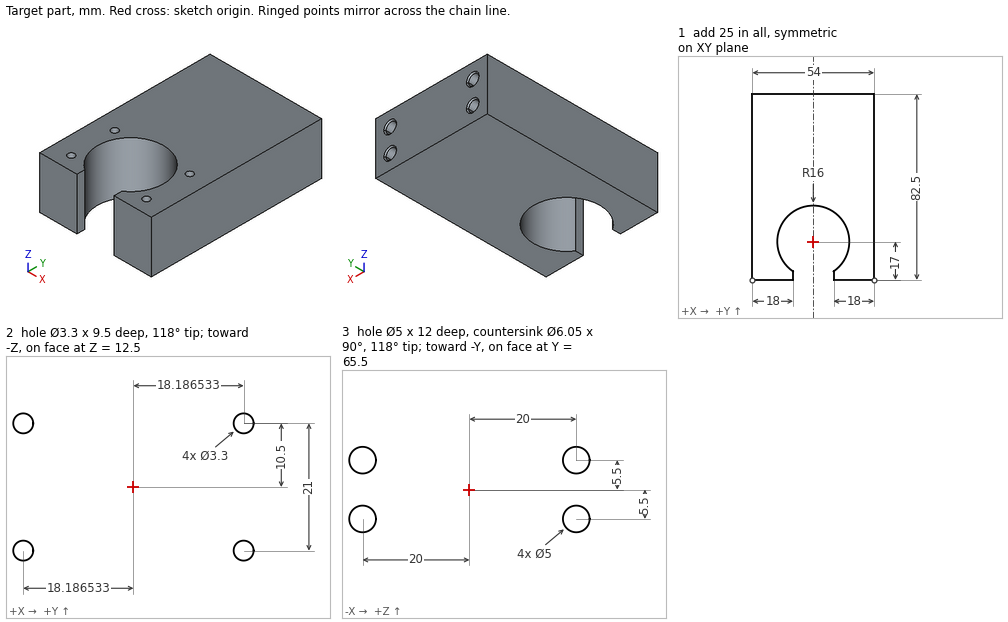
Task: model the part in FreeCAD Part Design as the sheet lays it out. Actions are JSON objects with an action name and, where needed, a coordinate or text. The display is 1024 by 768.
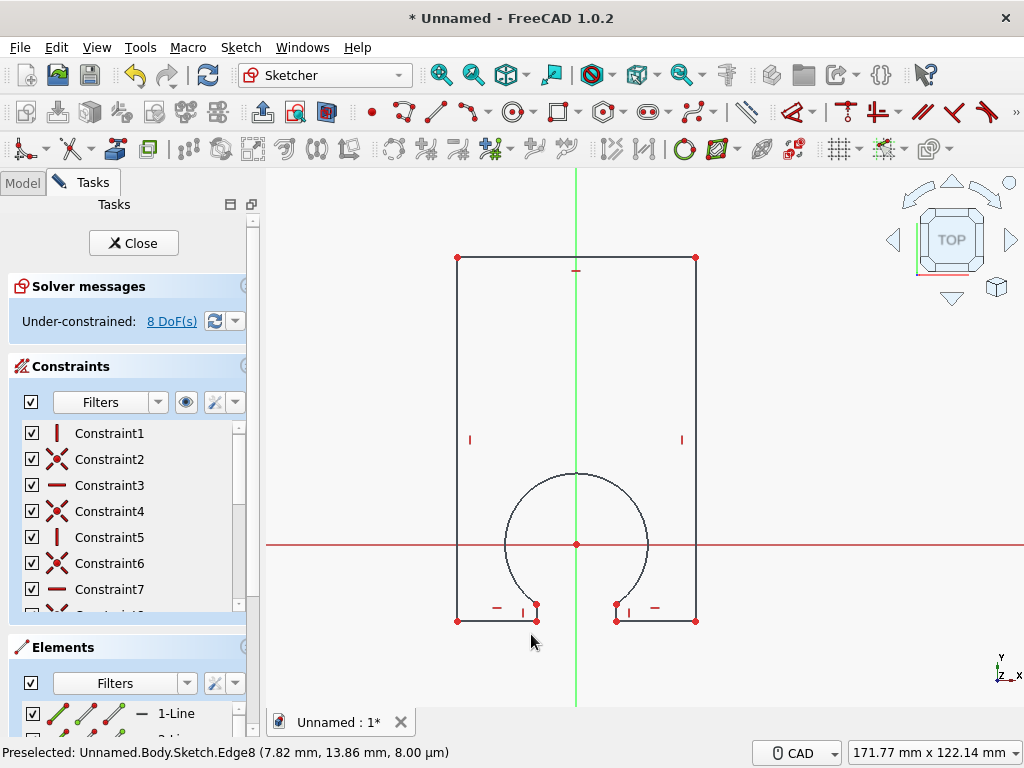
{"action": "left_click", "coordinate": [696, 621]}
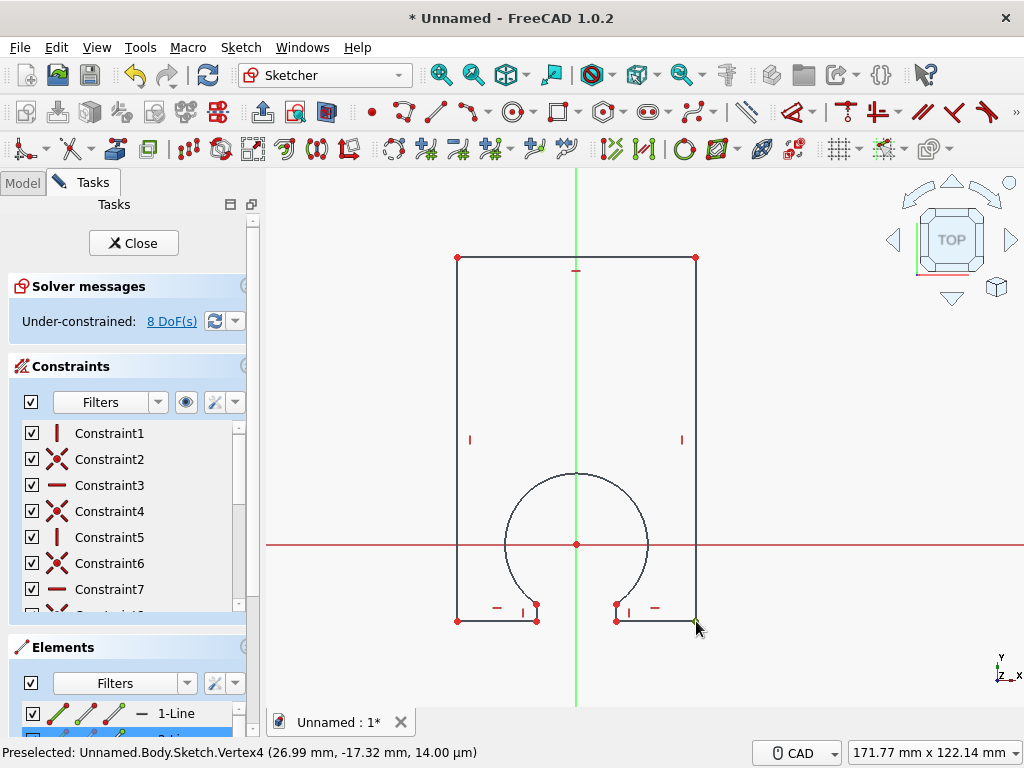
{"action": "left_click", "coordinate": [457, 621]}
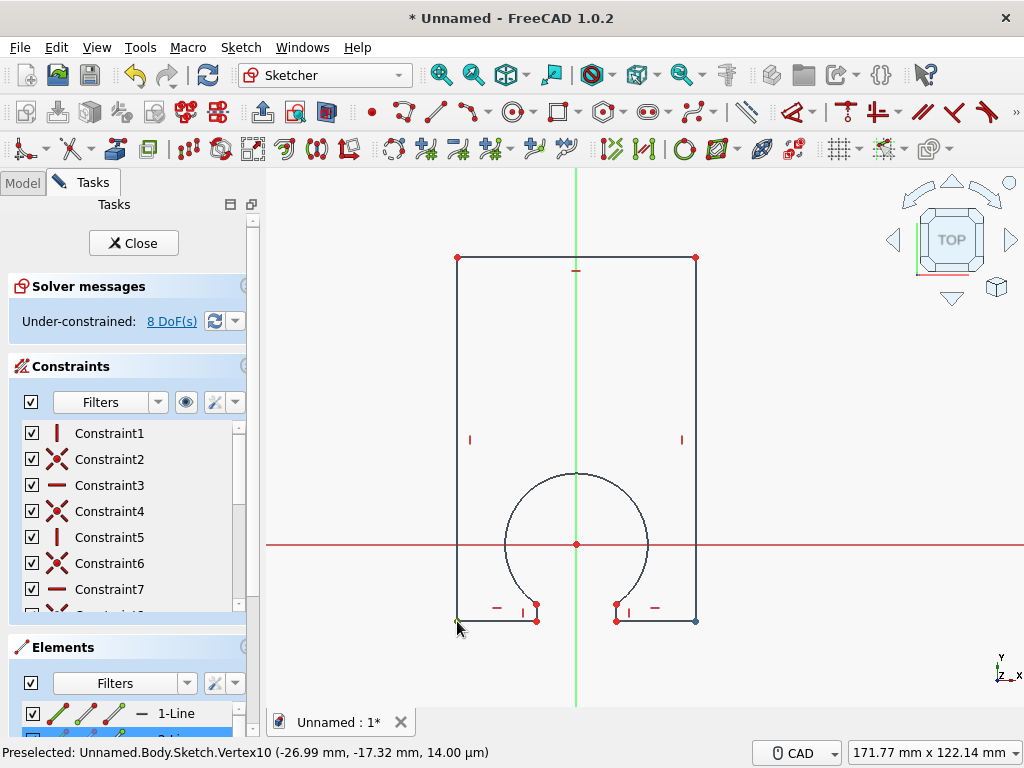
{"action": "left_click", "coordinate": [576, 644]}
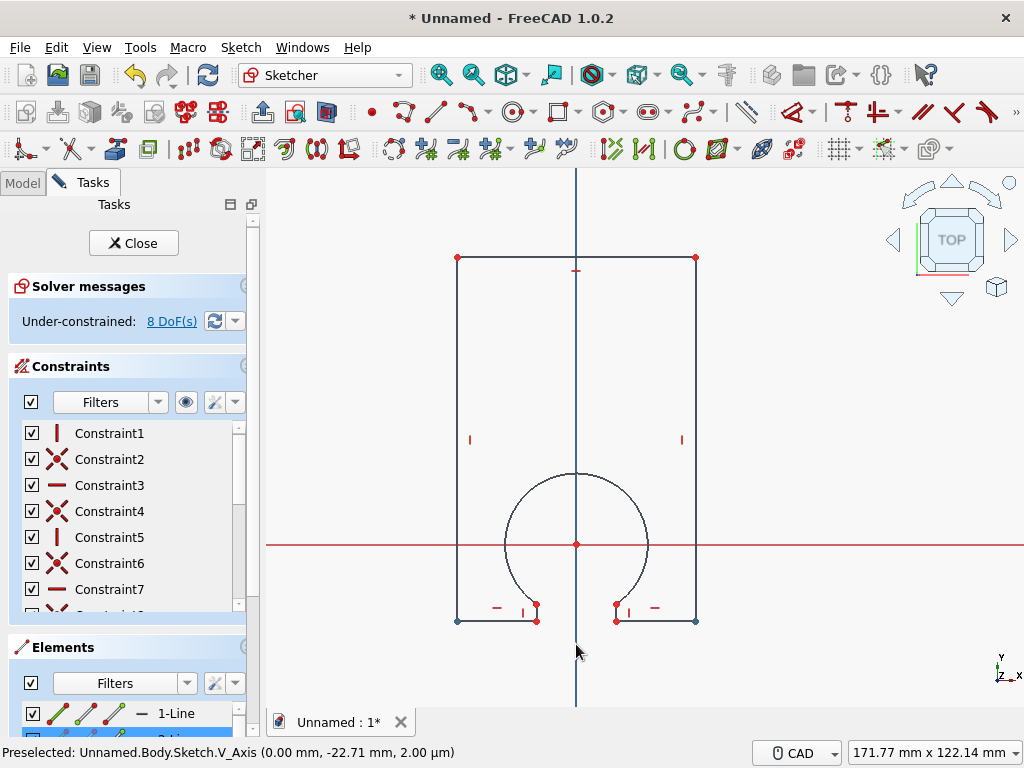
{"action": "key", "text": "s"}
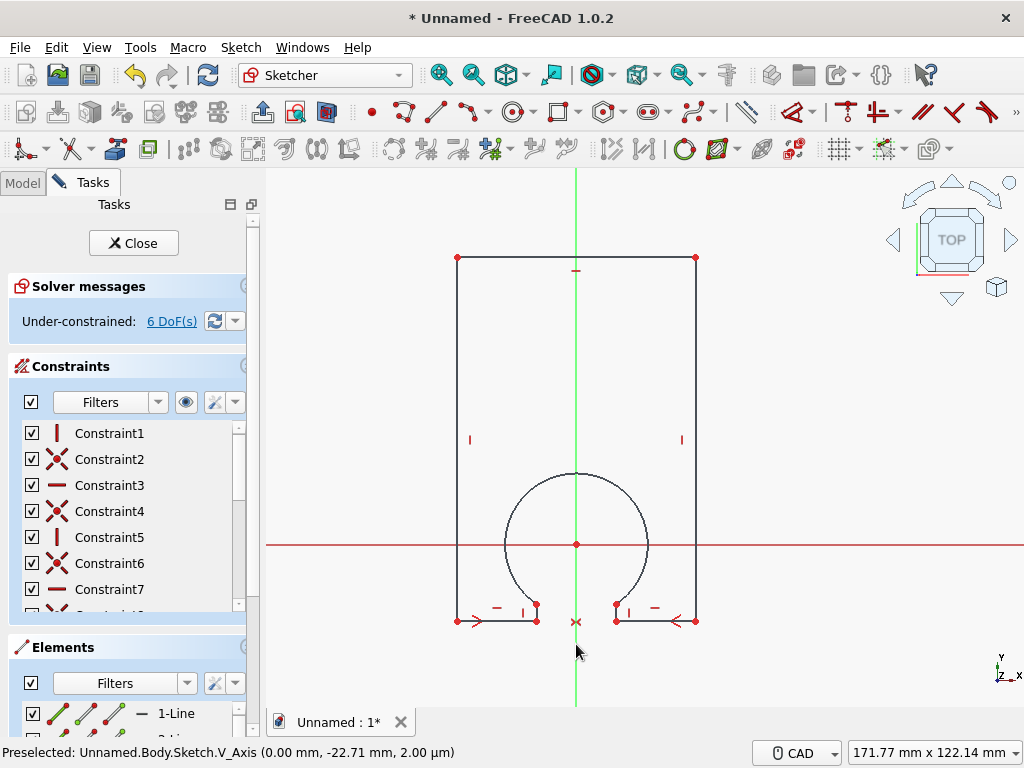
{"action": "left_click", "coordinate": [792, 112]}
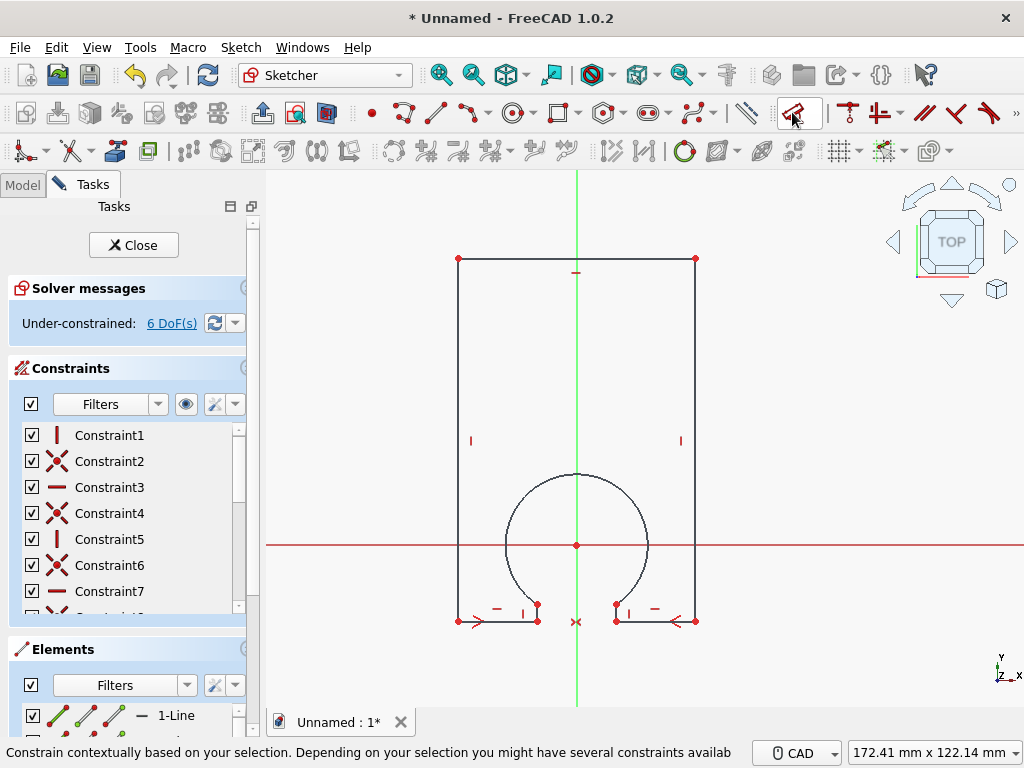
{"action": "left_click", "coordinate": [637, 508]}
{"action": "left_click", "coordinate": [664, 491]}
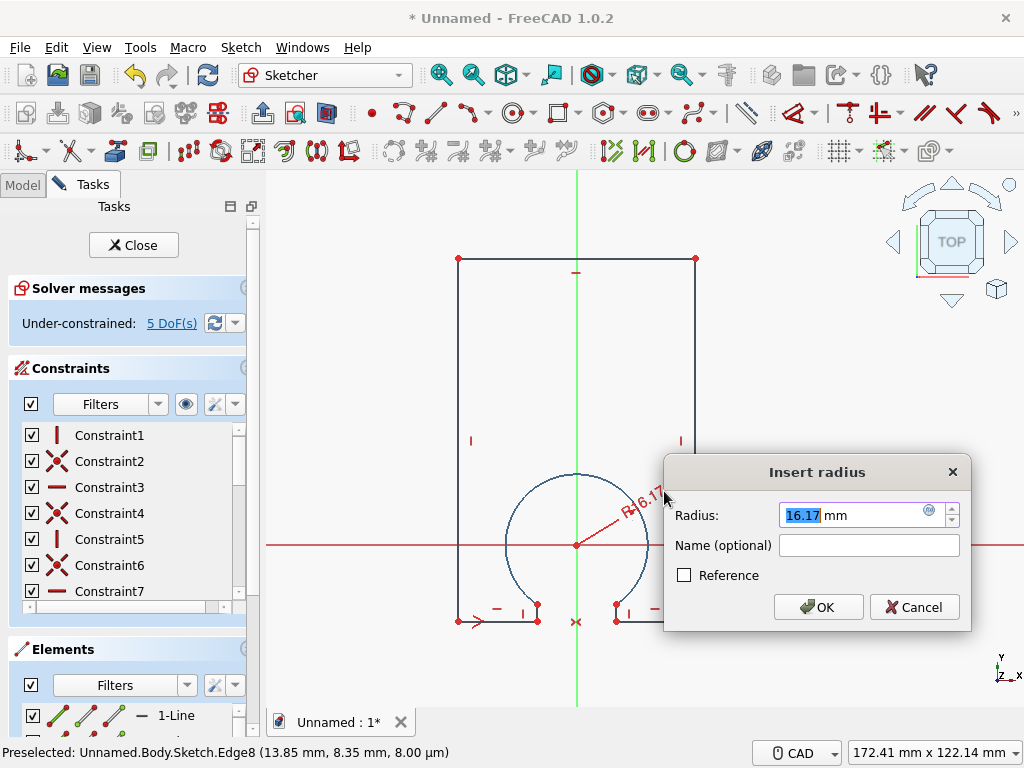
{"action": "type", "text": "16"}
{"action": "key", "text": "Return"}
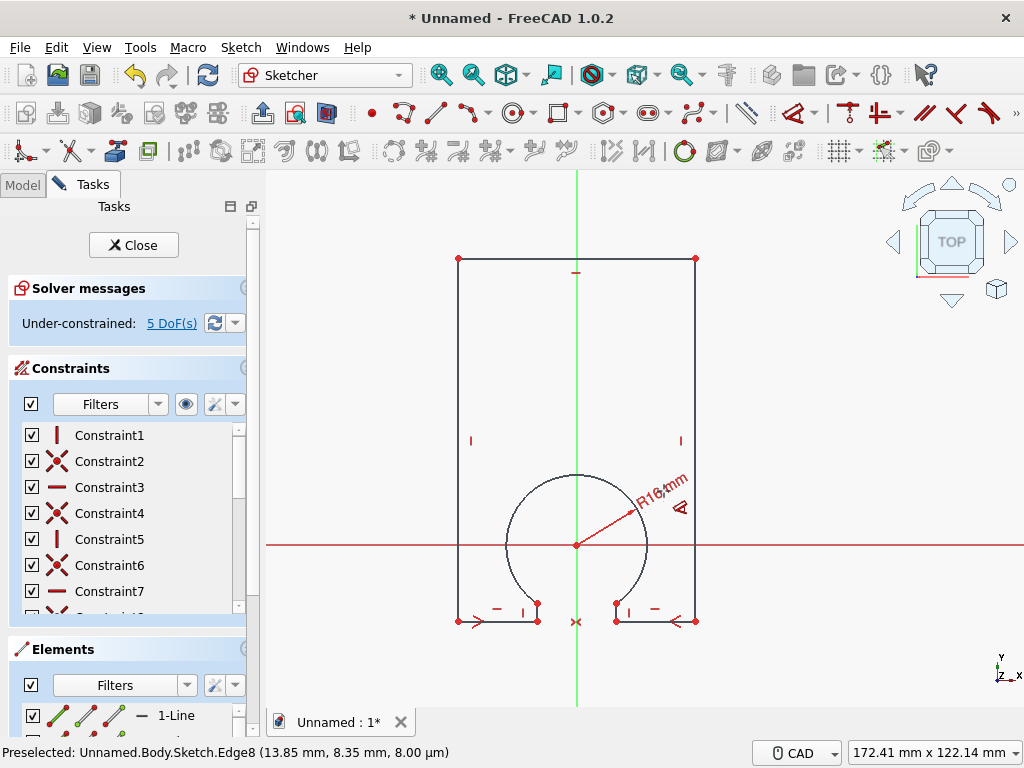
{"action": "left_click", "coordinate": [640, 622]}
{"action": "left_click", "coordinate": [656, 656]}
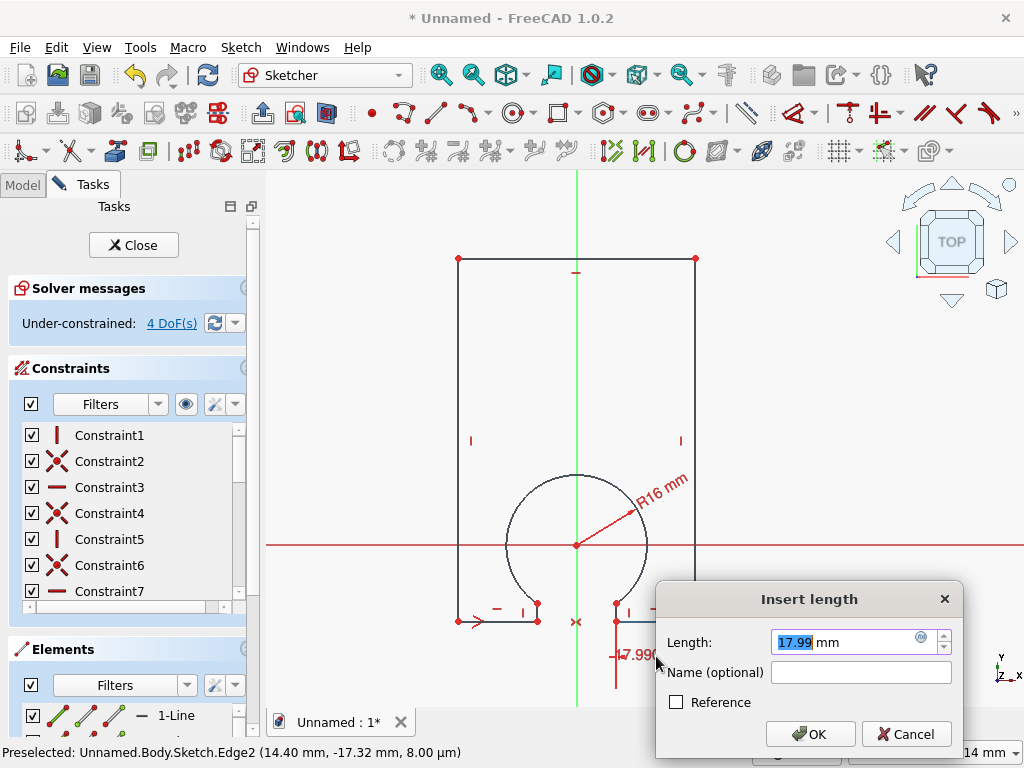
{"action": "type", "text": "18"}
{"action": "key", "text": "Return"}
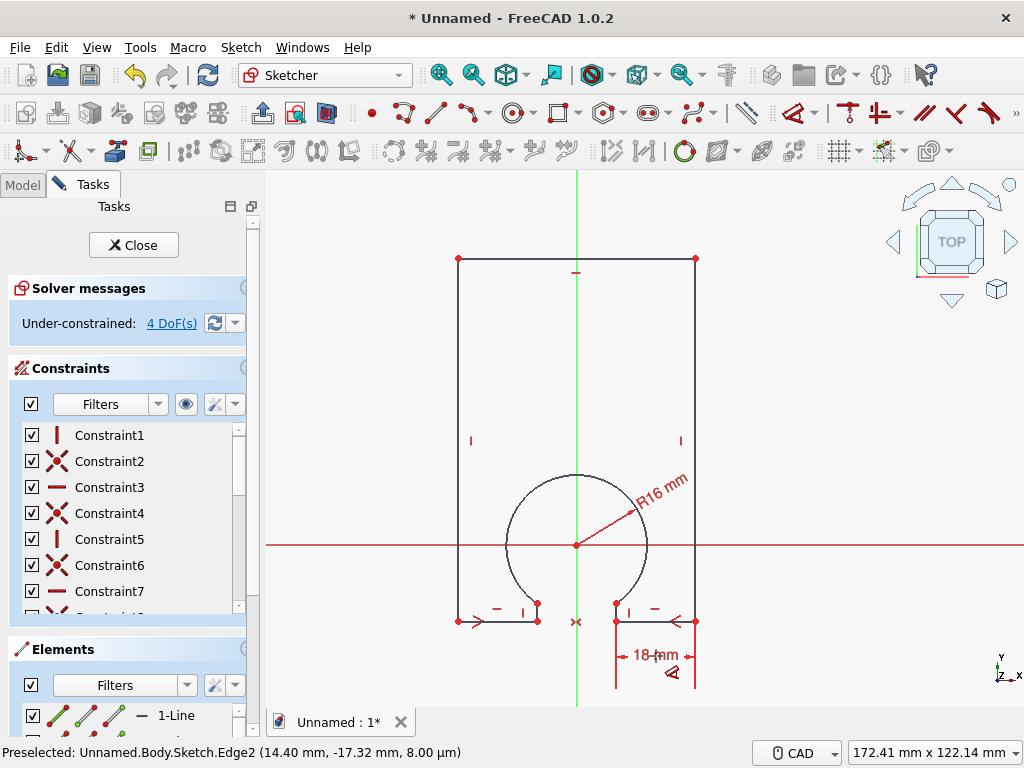
{"action": "left_click", "coordinate": [624, 259]}
{"action": "left_click", "coordinate": [522, 225]}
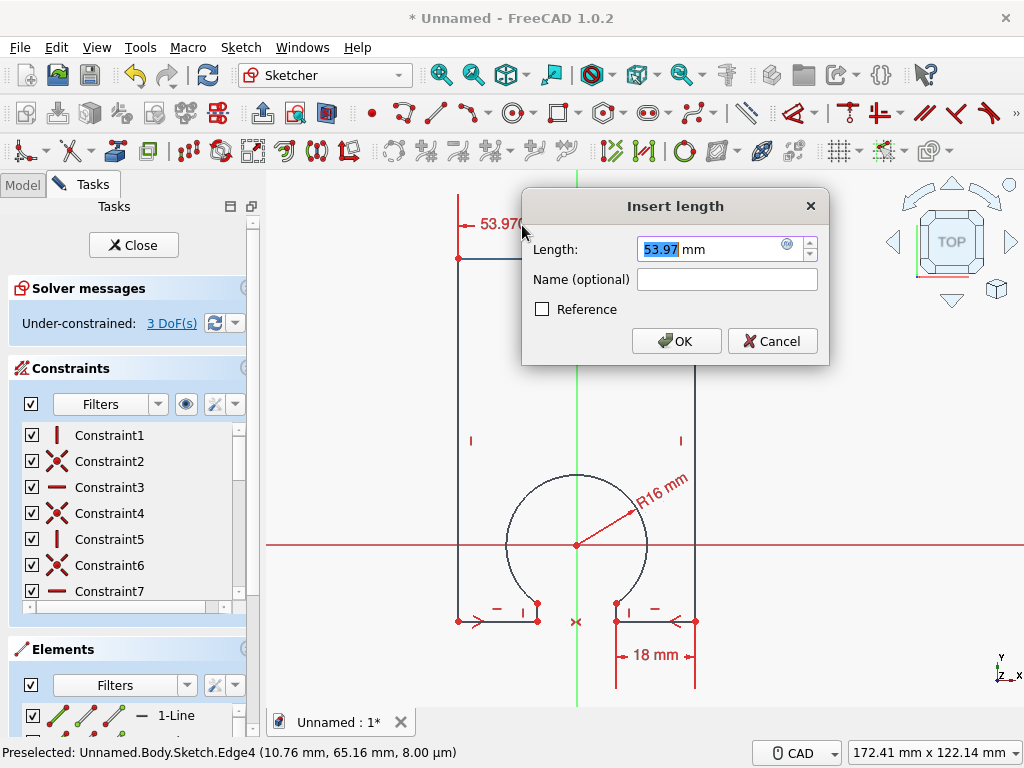
{"action": "type", "text": "54"}
{"action": "key", "text": "Return"}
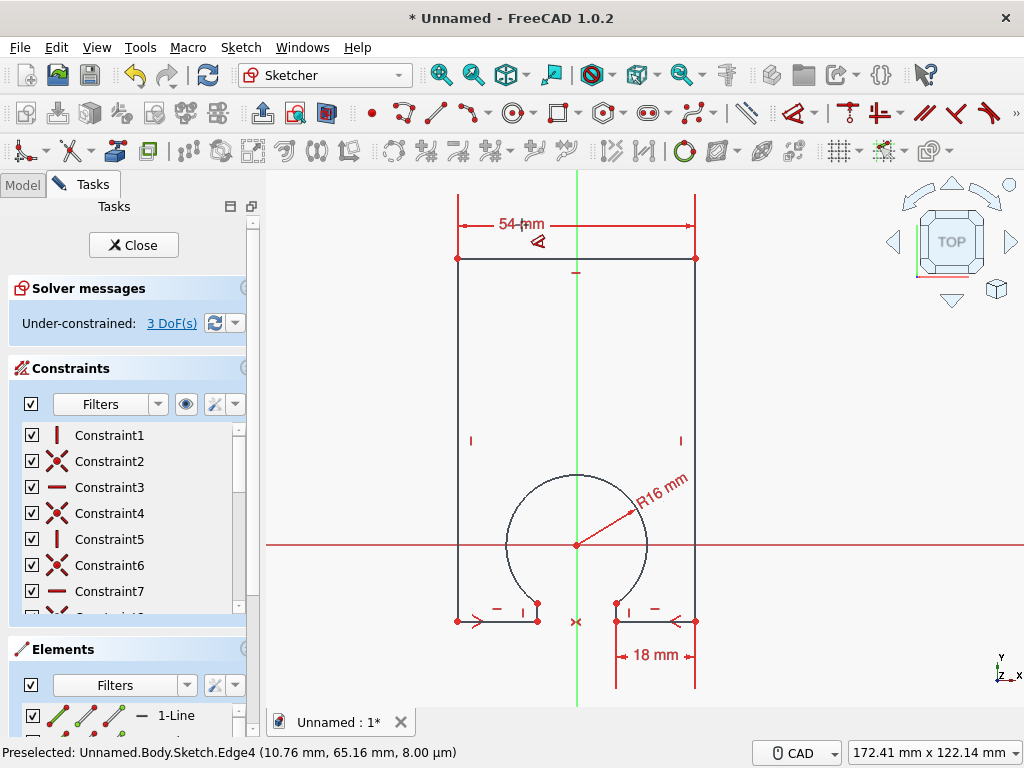
{"action": "left_click", "coordinate": [482, 622]}
{"action": "left_click", "coordinate": [498, 656]}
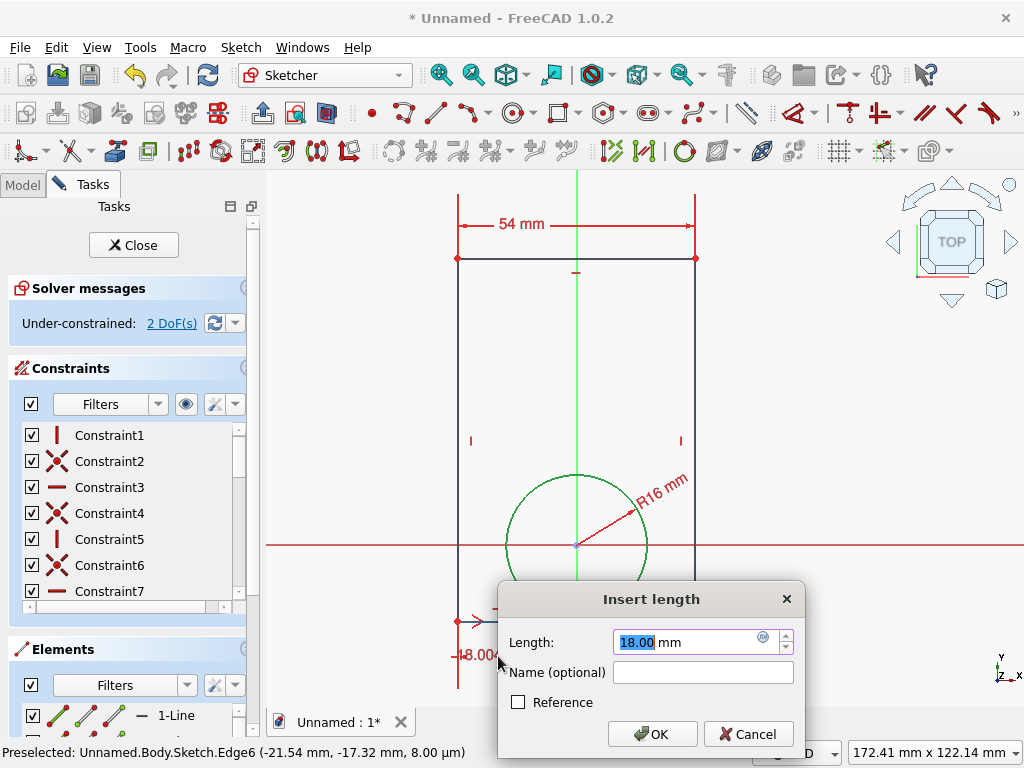
{"action": "type", "text": "18"}
{"action": "key", "text": "Return"}